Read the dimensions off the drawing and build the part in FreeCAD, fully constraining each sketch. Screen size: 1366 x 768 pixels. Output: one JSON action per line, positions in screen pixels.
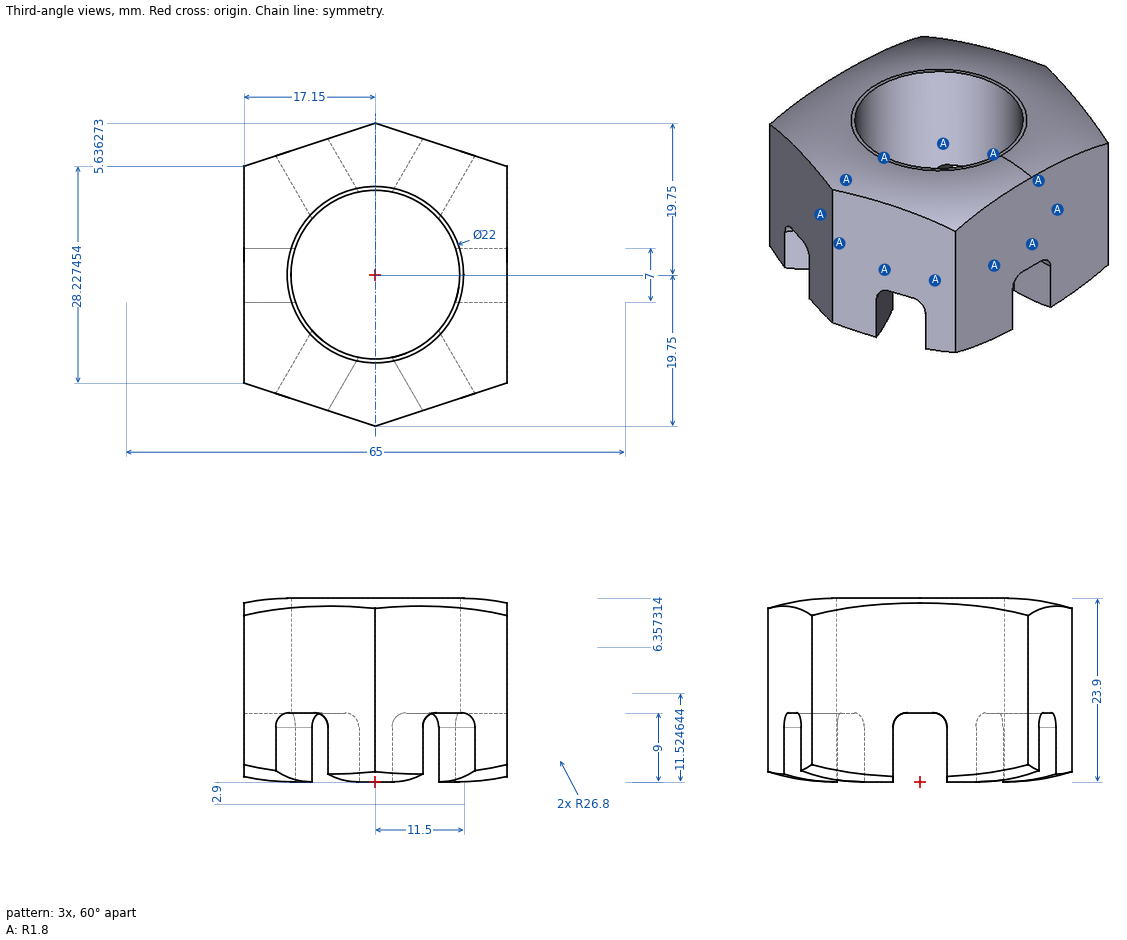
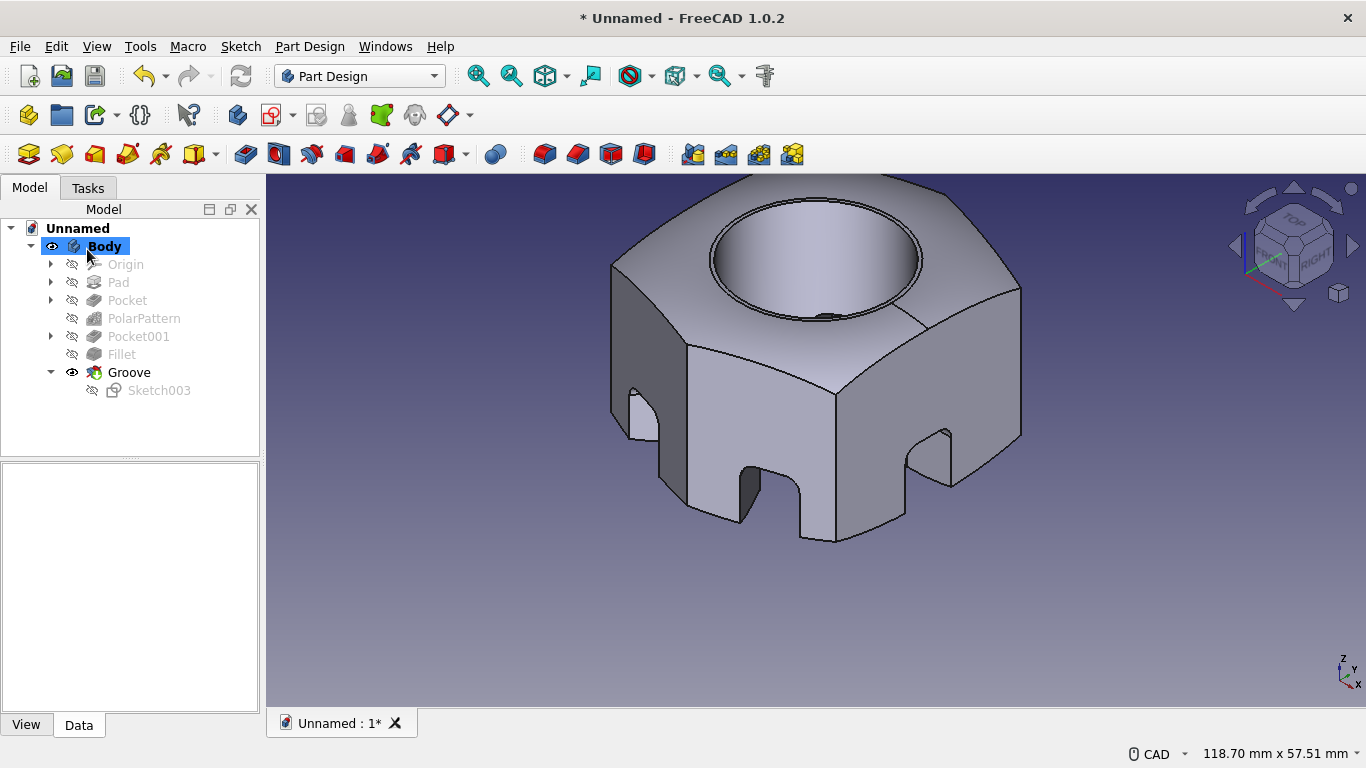
{"action": "left_click", "coordinate": [479, 76]}